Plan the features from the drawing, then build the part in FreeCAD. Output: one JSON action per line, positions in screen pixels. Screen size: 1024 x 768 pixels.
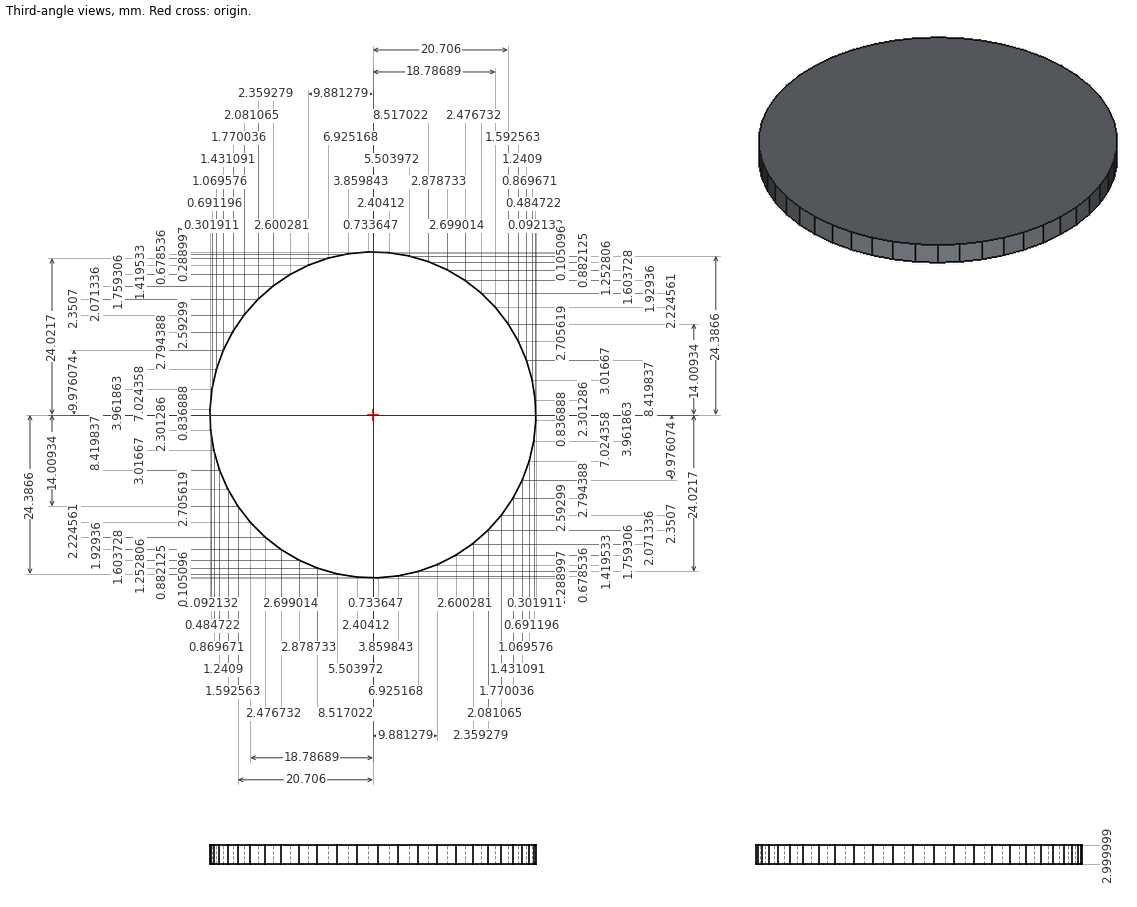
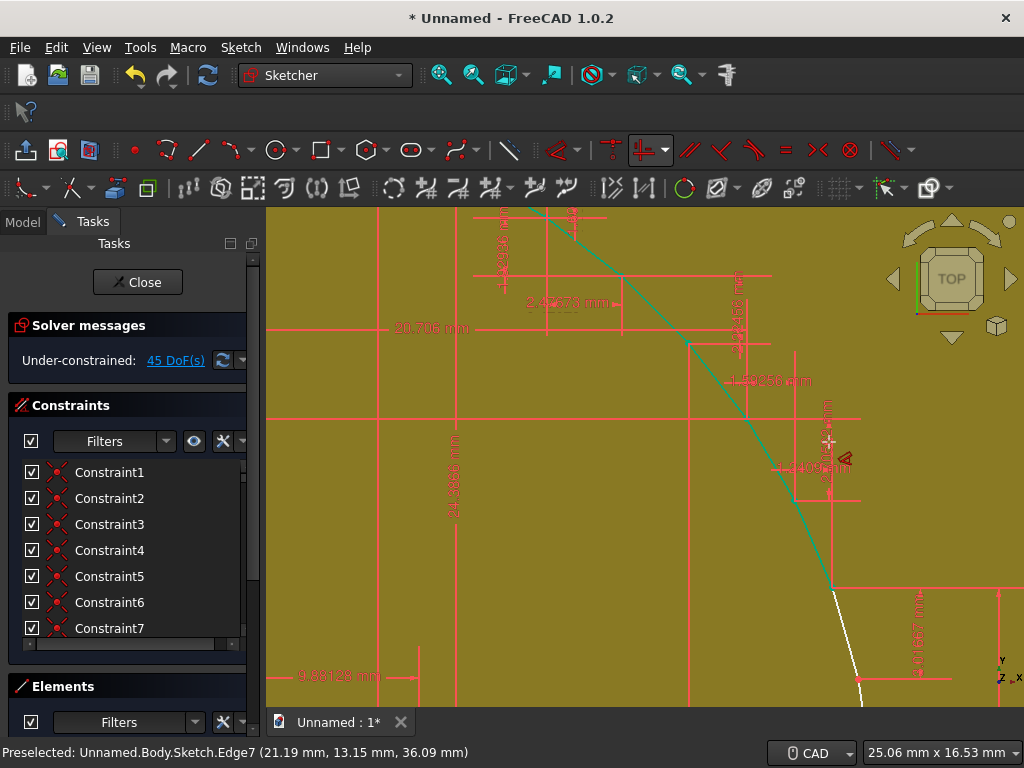
{"action": "scroll", "coordinate": [840, 615], "scroll_direction": "up", "scroll_amount": 3}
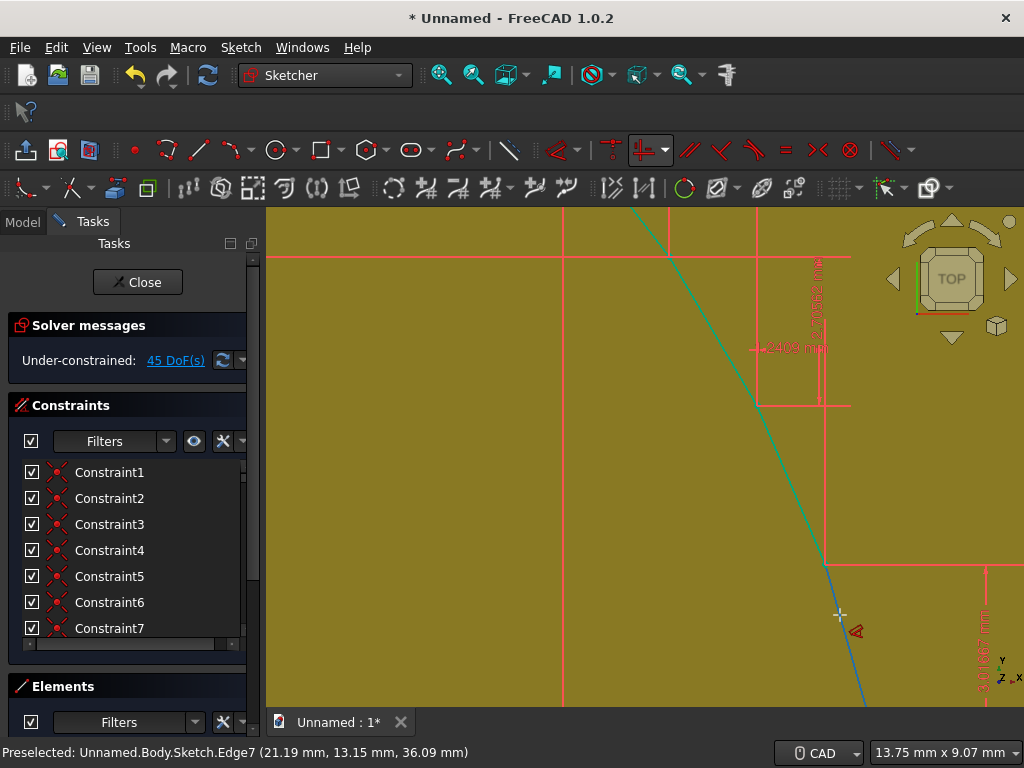
{"action": "left_click", "coordinate": [840, 615]}
{"action": "left_click", "coordinate": [842, 531]}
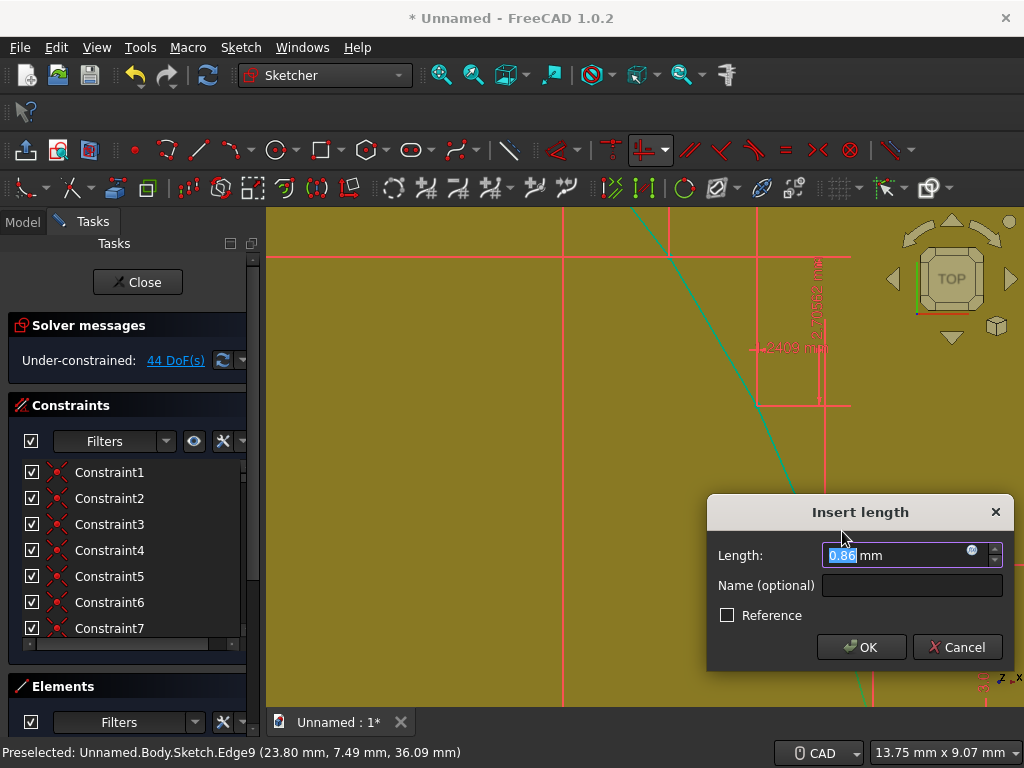
{"action": "type", "text": "0.869671"}
{"action": "key", "text": "Return"}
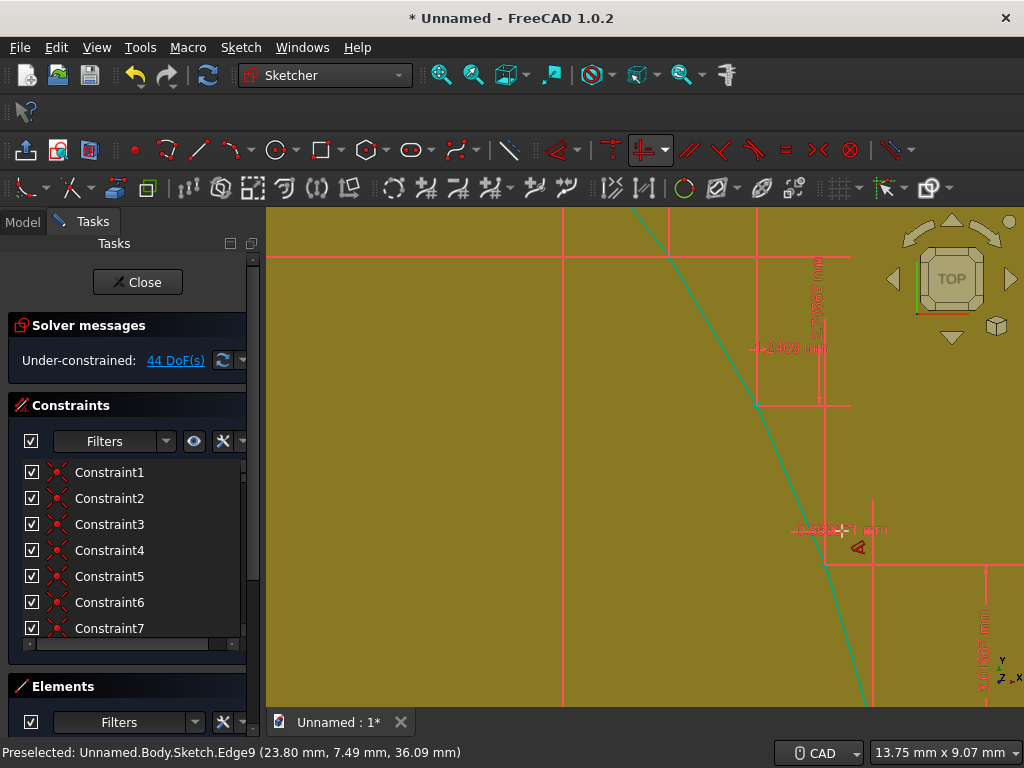
{"action": "scroll", "coordinate": [707, 386], "scroll_direction": "down", "scroll_amount": 11}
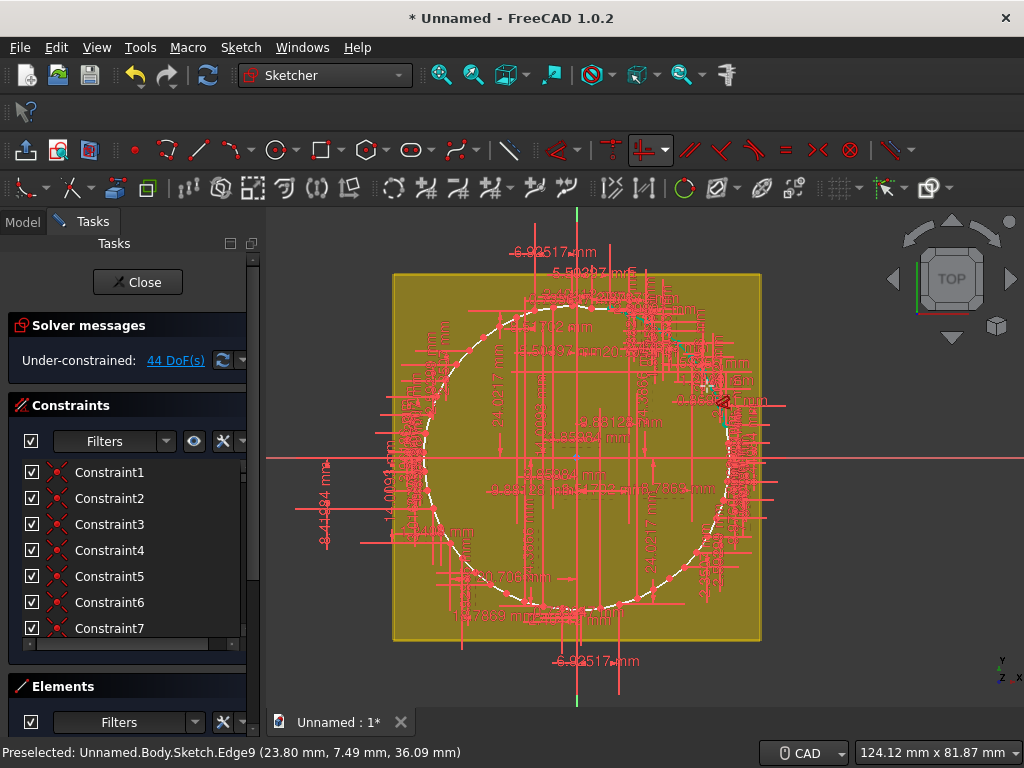
{"action": "scroll", "coordinate": [727, 430], "scroll_direction": "up", "scroll_amount": 13}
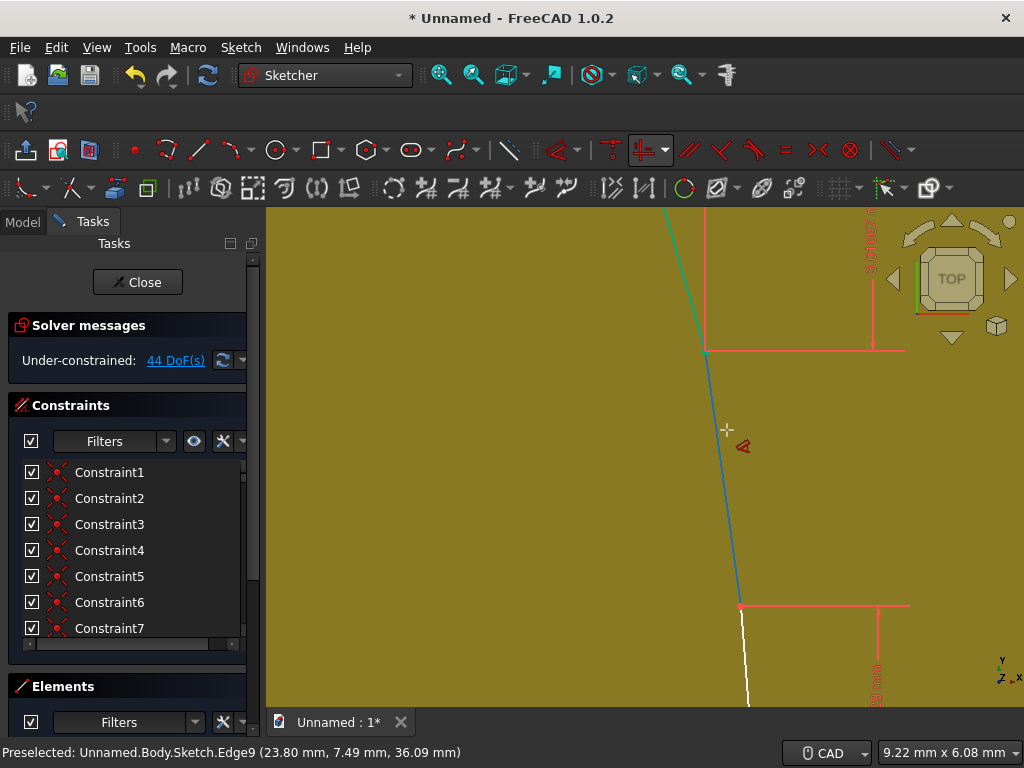
{"action": "left_click", "coordinate": [716, 428]}
{"action": "left_click", "coordinate": [723, 317]}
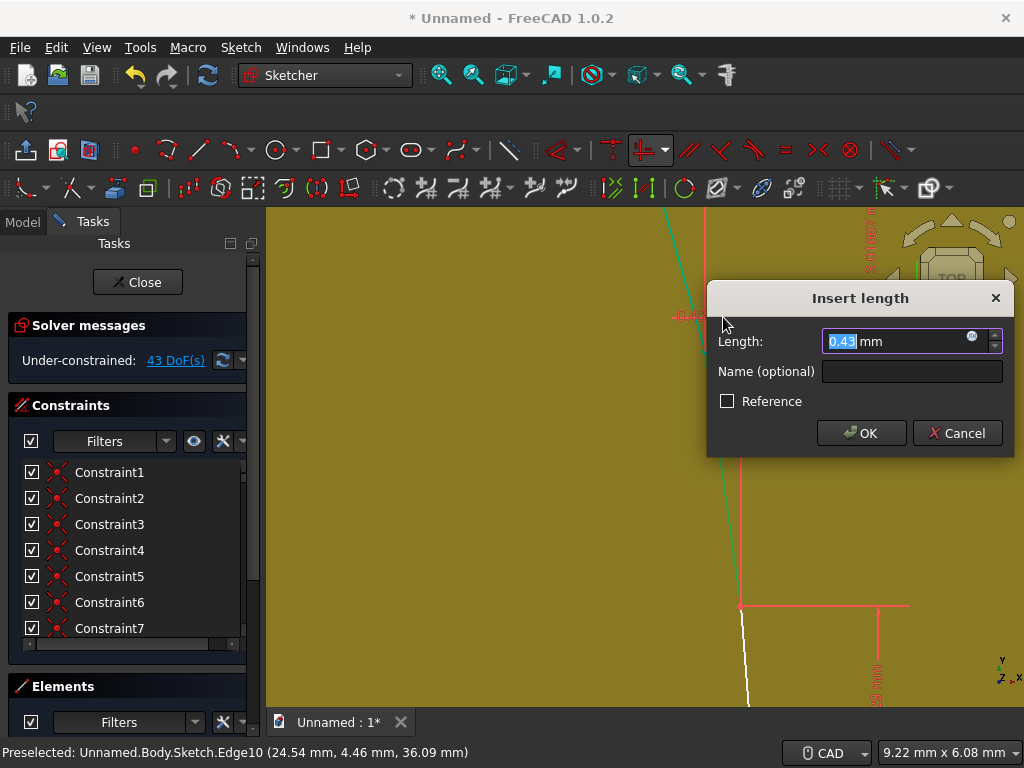
{"action": "type", "text": "0.484722"}
{"action": "key", "text": "Return"}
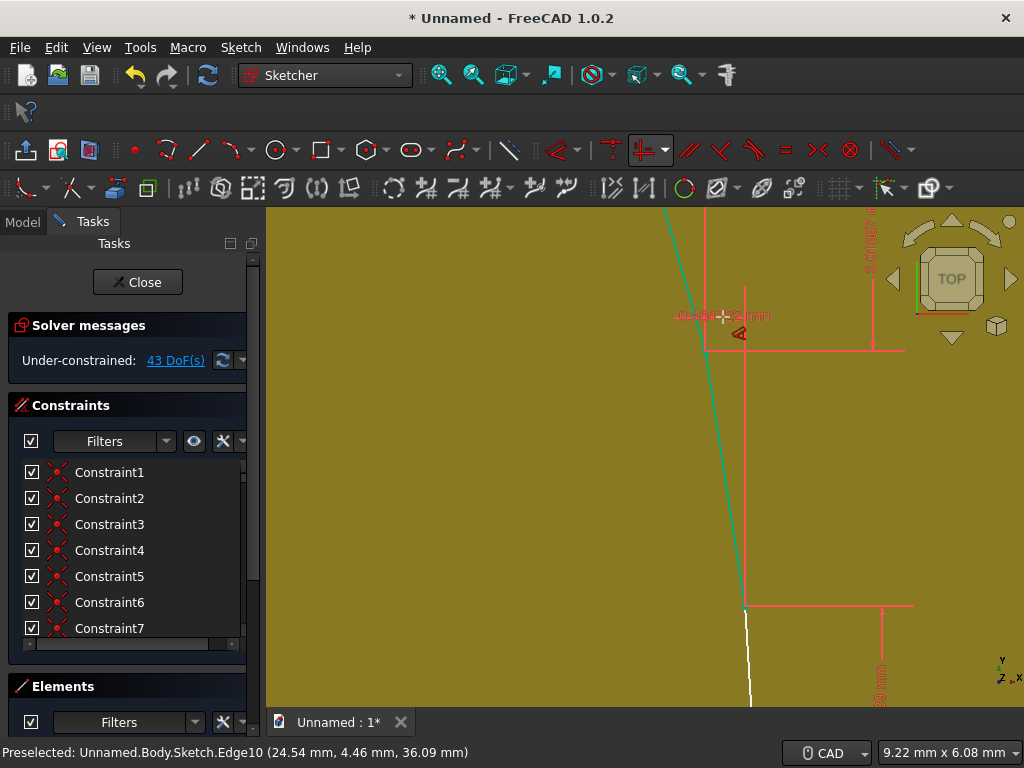
{"action": "scroll", "coordinate": [748, 658], "scroll_direction": "up", "scroll_amount": 9}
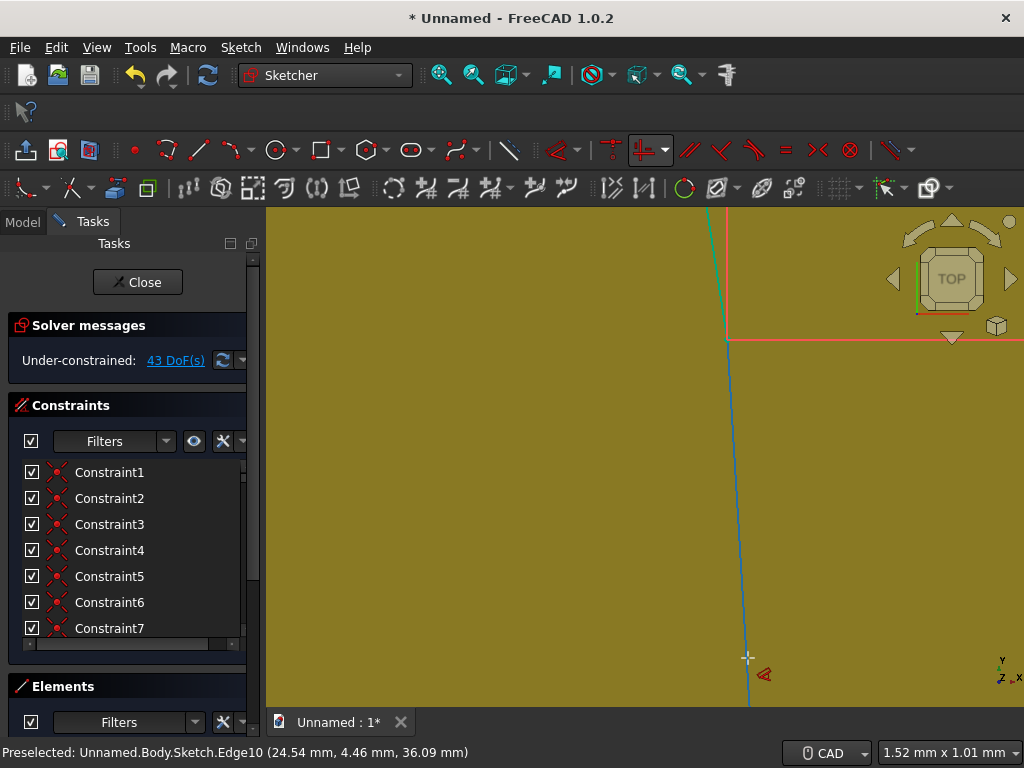
{"action": "left_click", "coordinate": [746, 652]}
{"action": "left_click", "coordinate": [775, 306]}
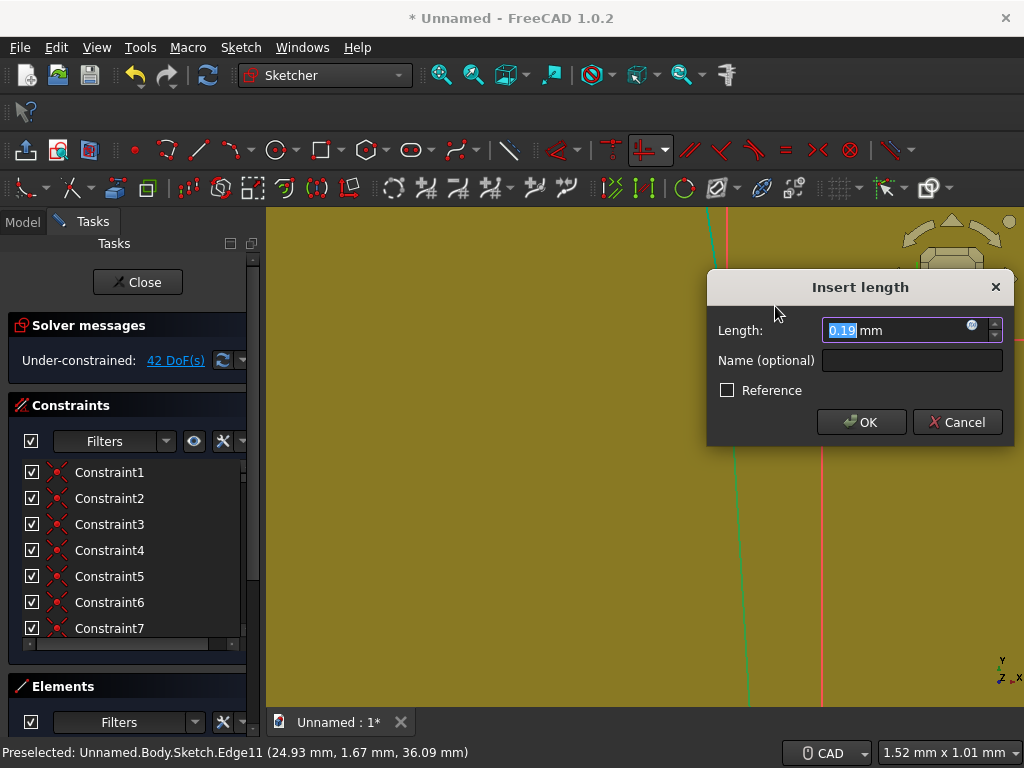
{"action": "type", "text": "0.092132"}
{"action": "key", "text": "Return"}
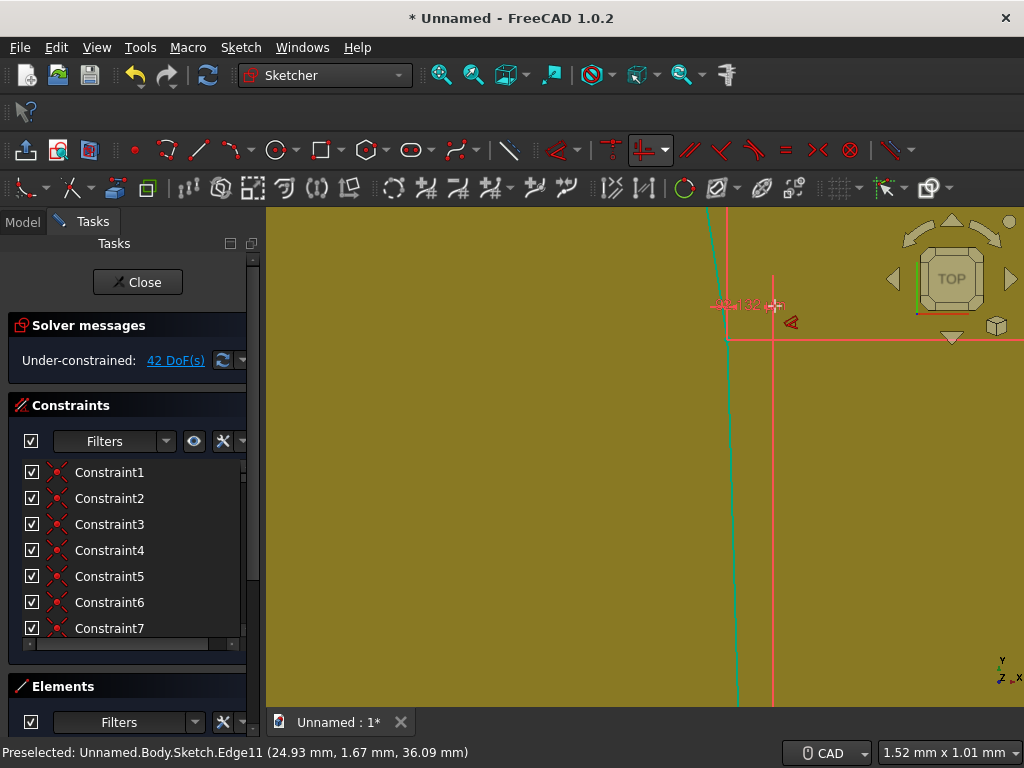
{"action": "scroll", "coordinate": [576, 457], "scroll_direction": "down", "scroll_amount": 15}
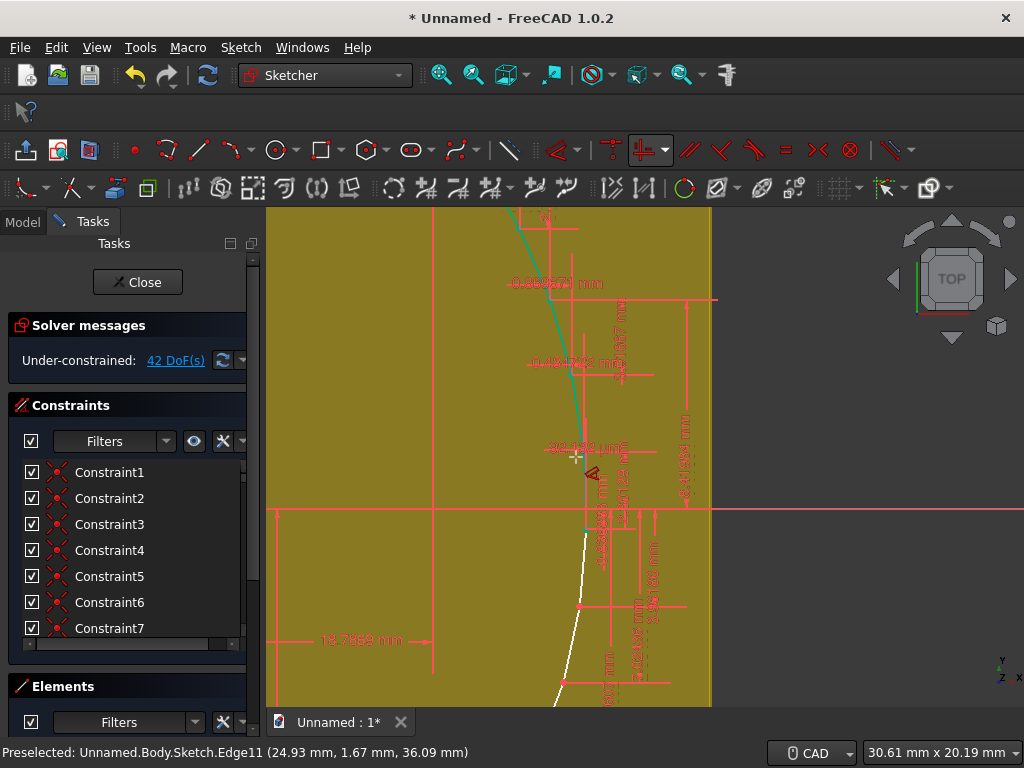
{"action": "scroll", "coordinate": [776, 440], "scroll_direction": "down", "scroll_amount": 7}